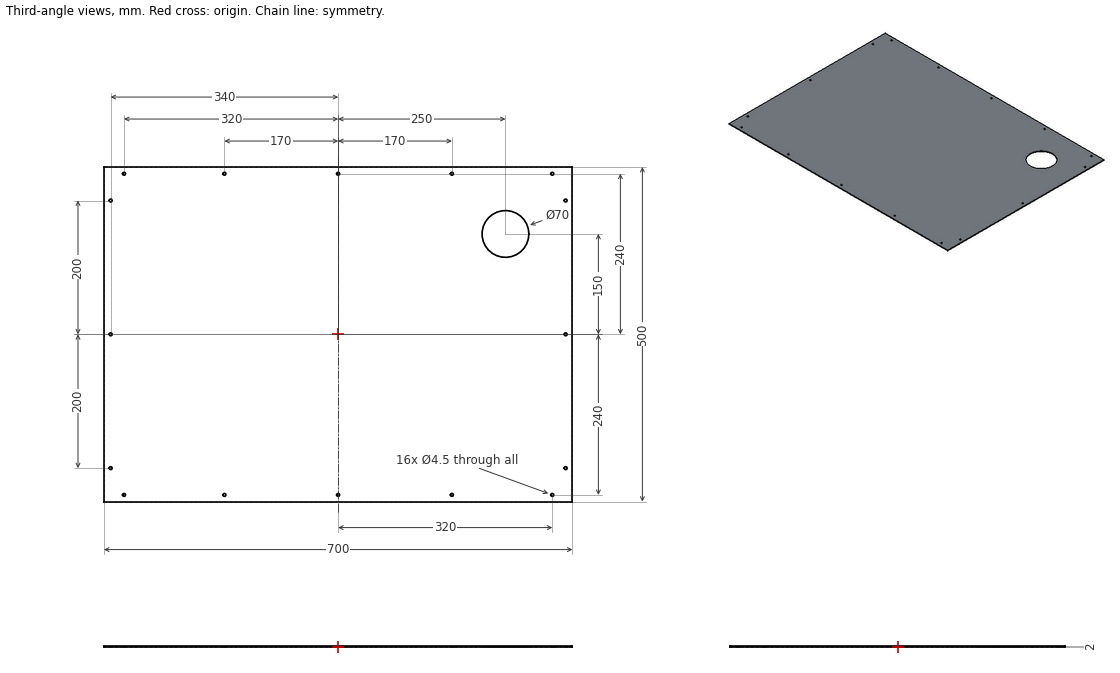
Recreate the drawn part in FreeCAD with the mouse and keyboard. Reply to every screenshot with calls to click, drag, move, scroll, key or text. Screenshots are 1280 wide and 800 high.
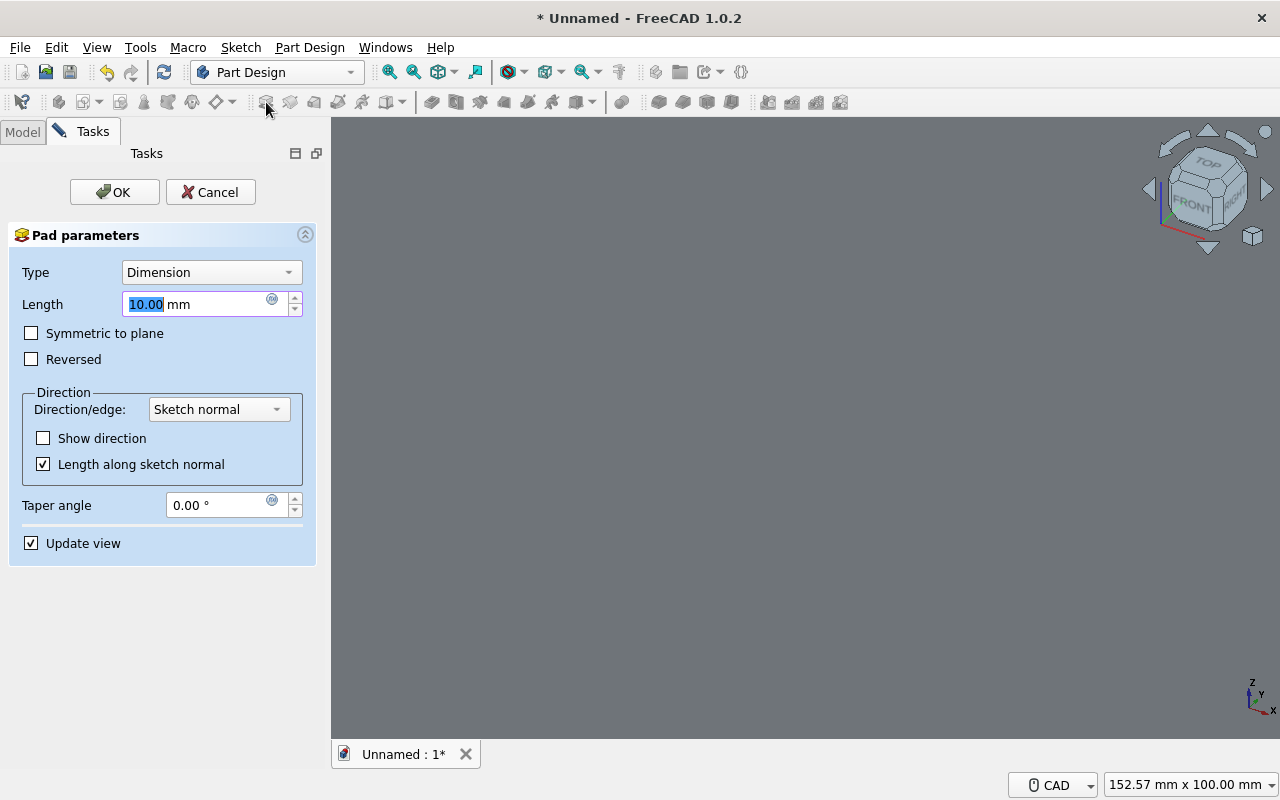
text(2)
key(Tab)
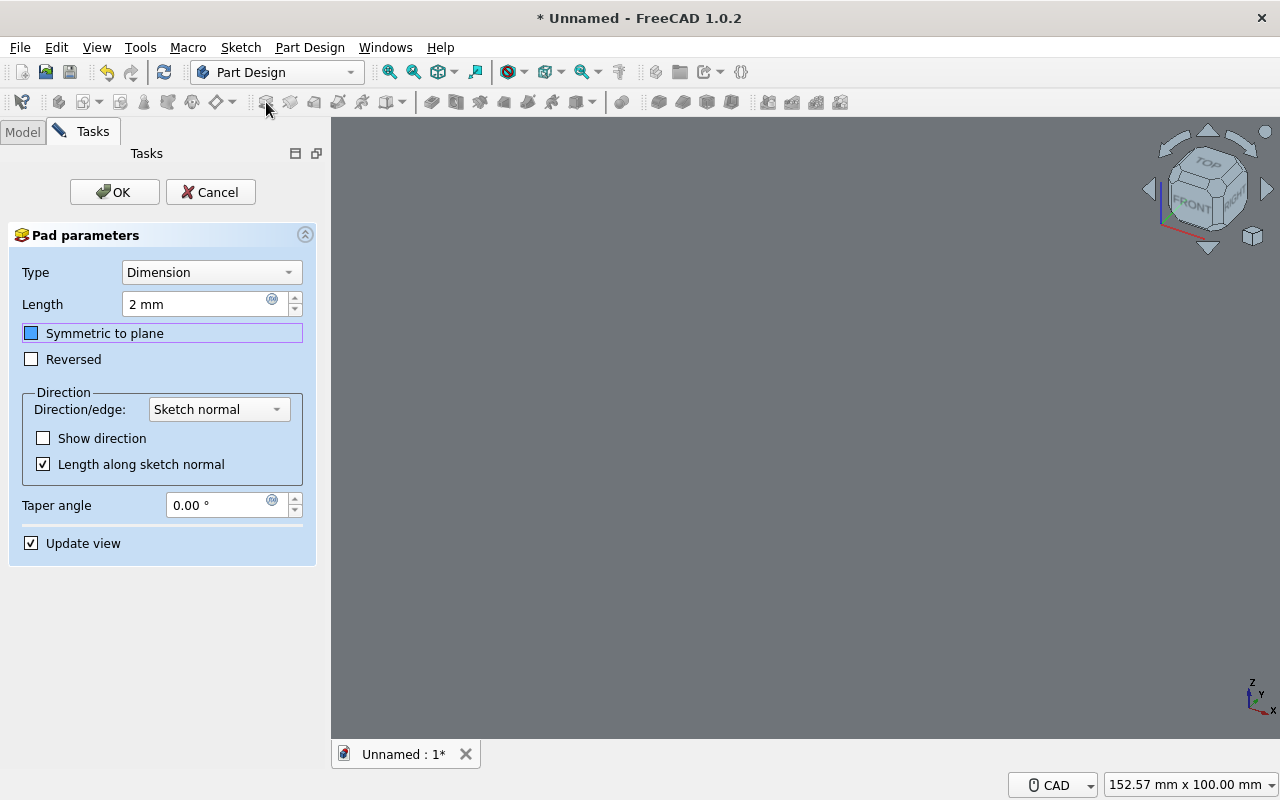
click(115, 192)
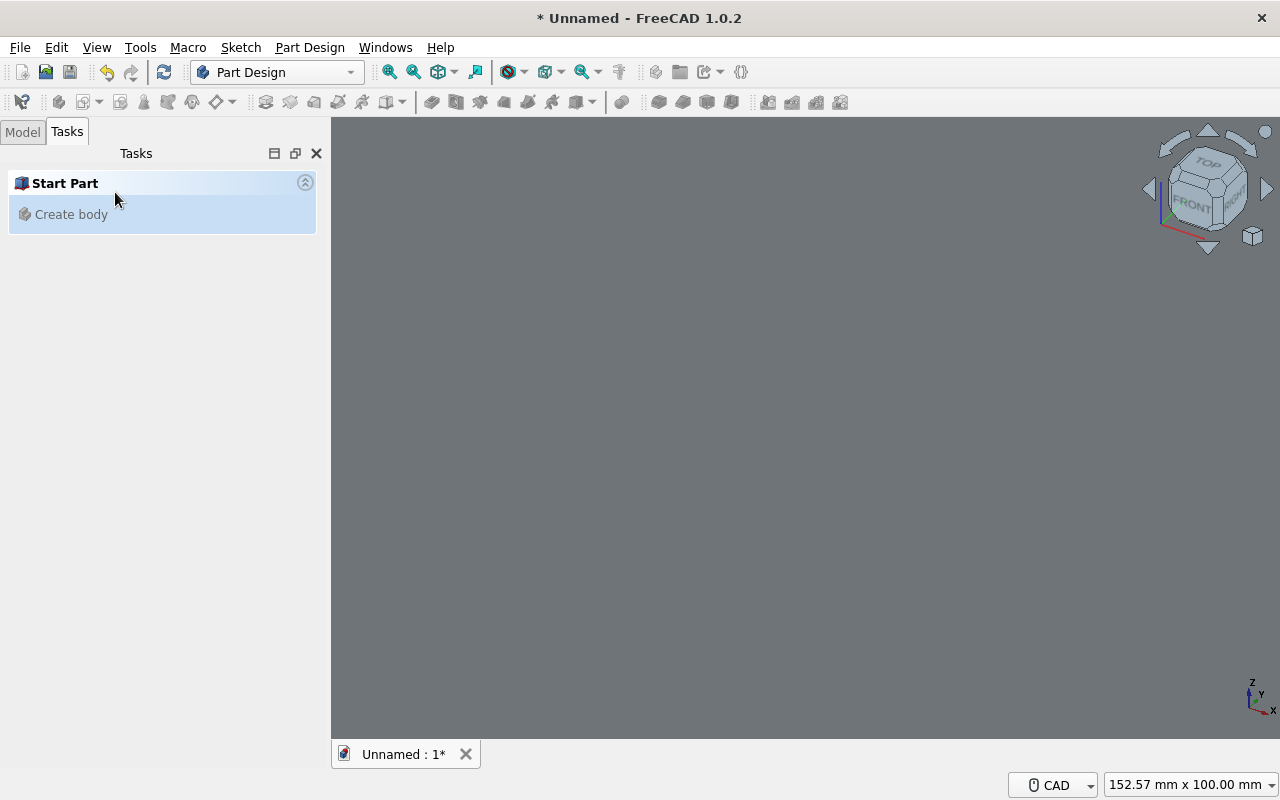
key(v)
key(f)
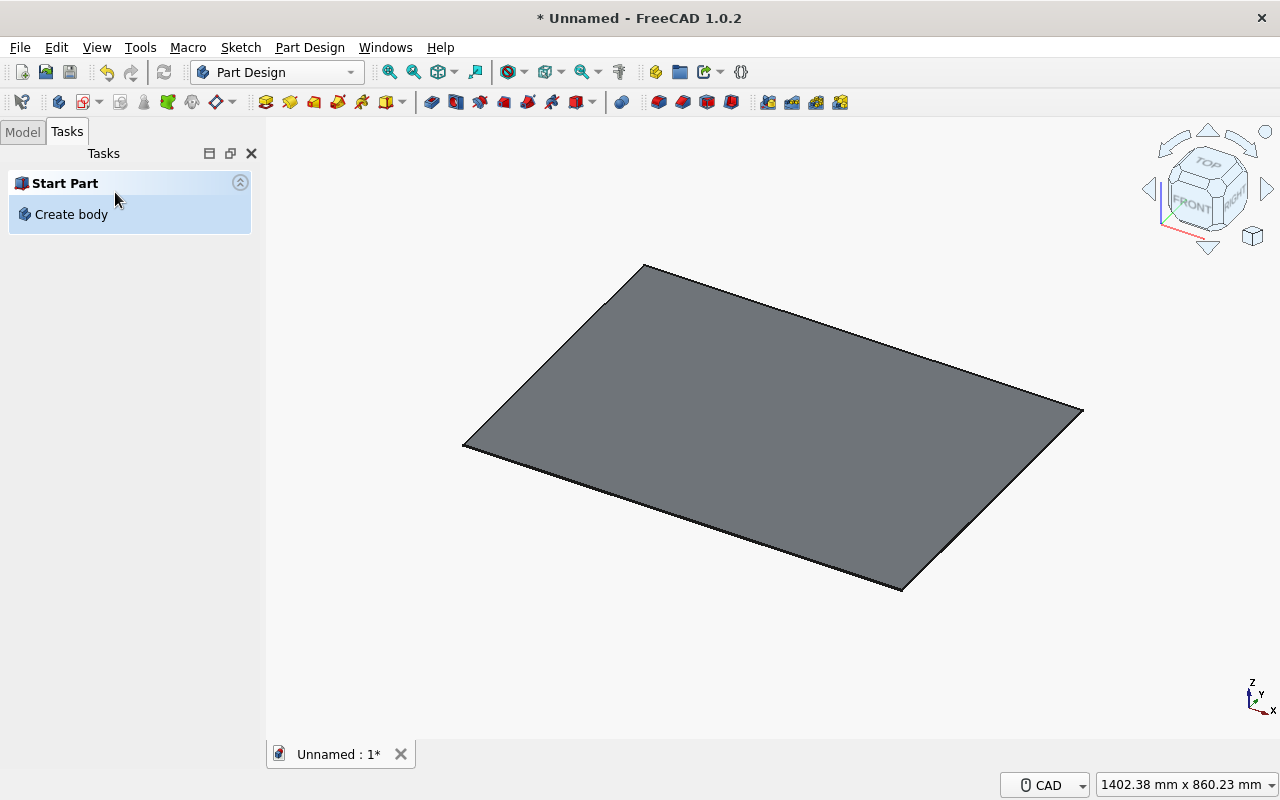
click(836, 447)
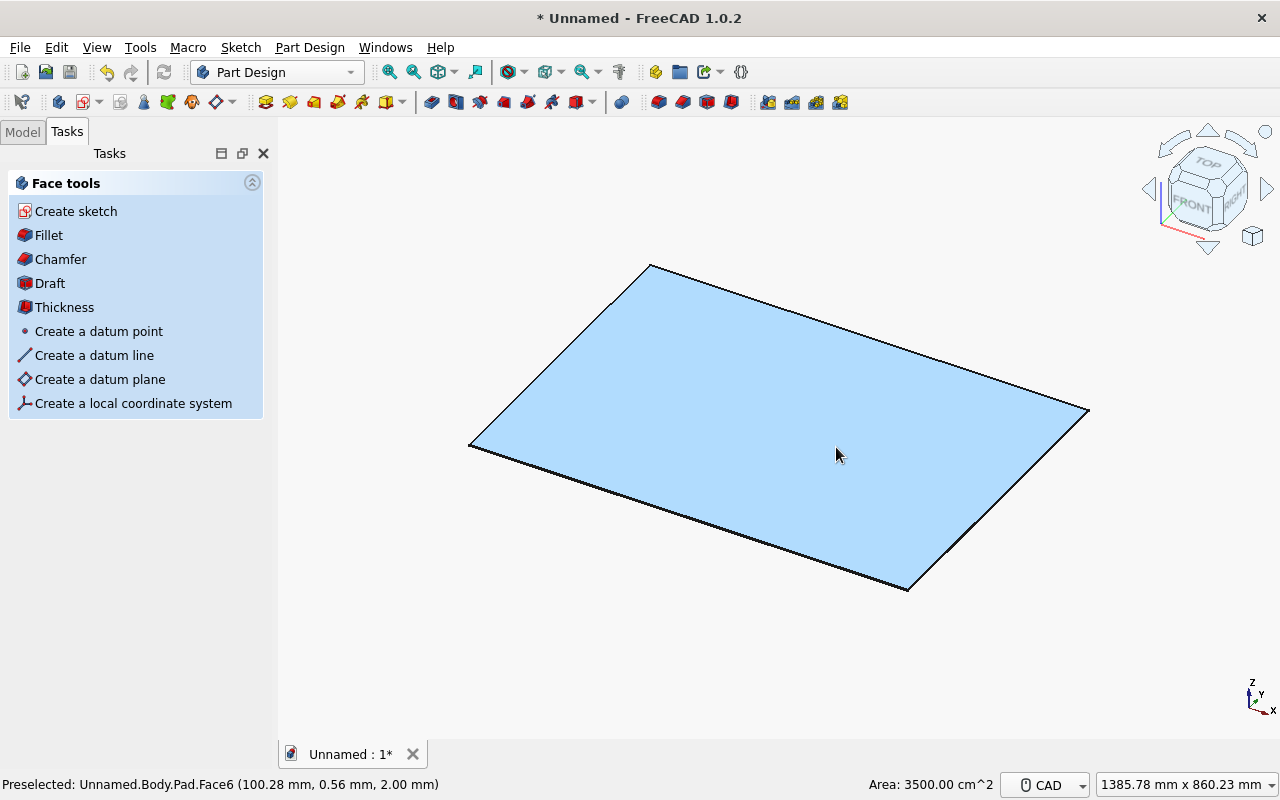
click(84, 102)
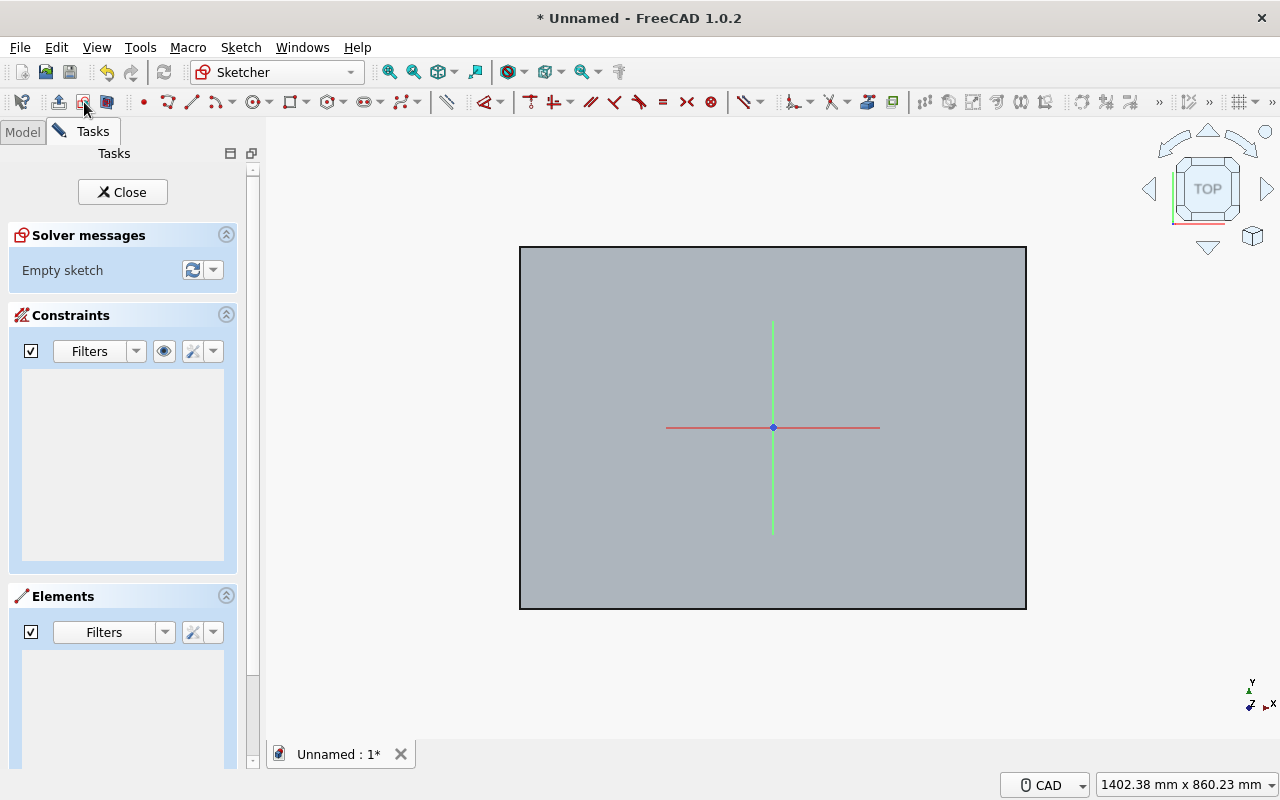
key(g)
key(c)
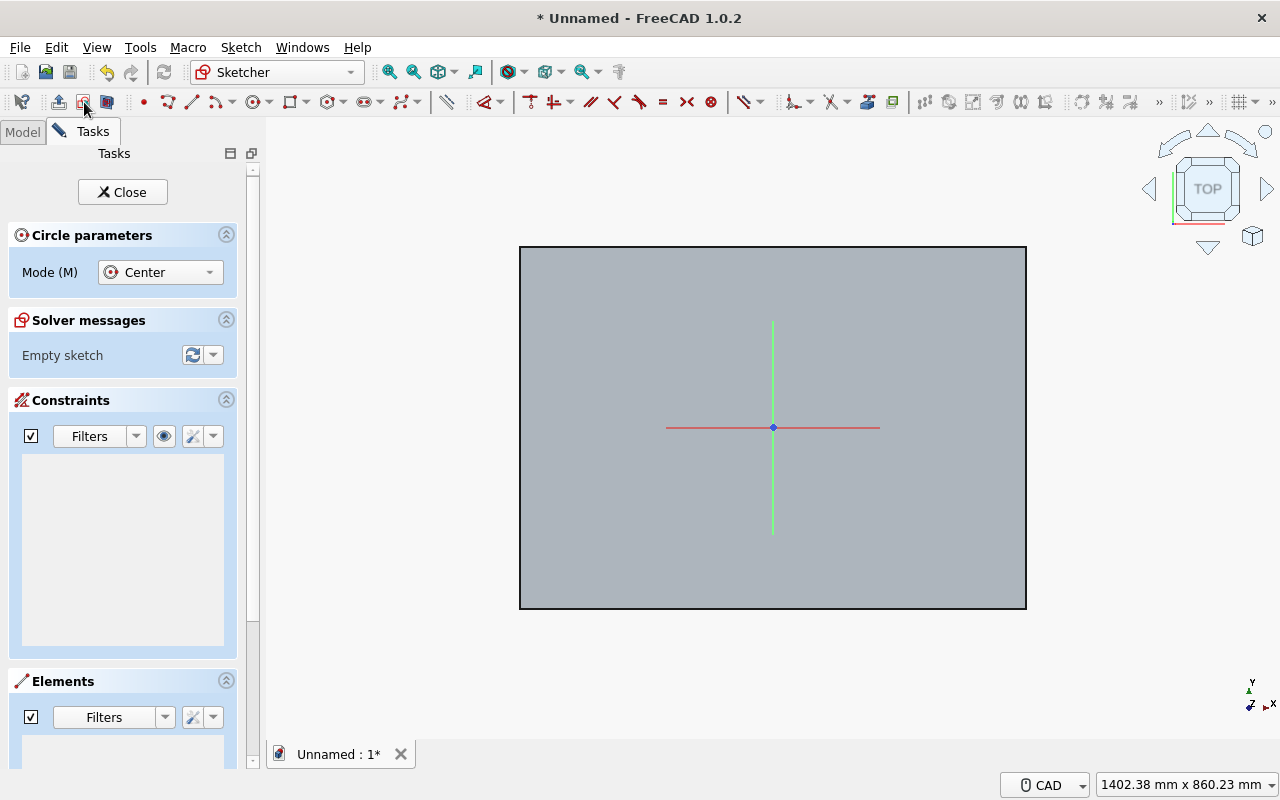
scroll(1004, 602, up, 14)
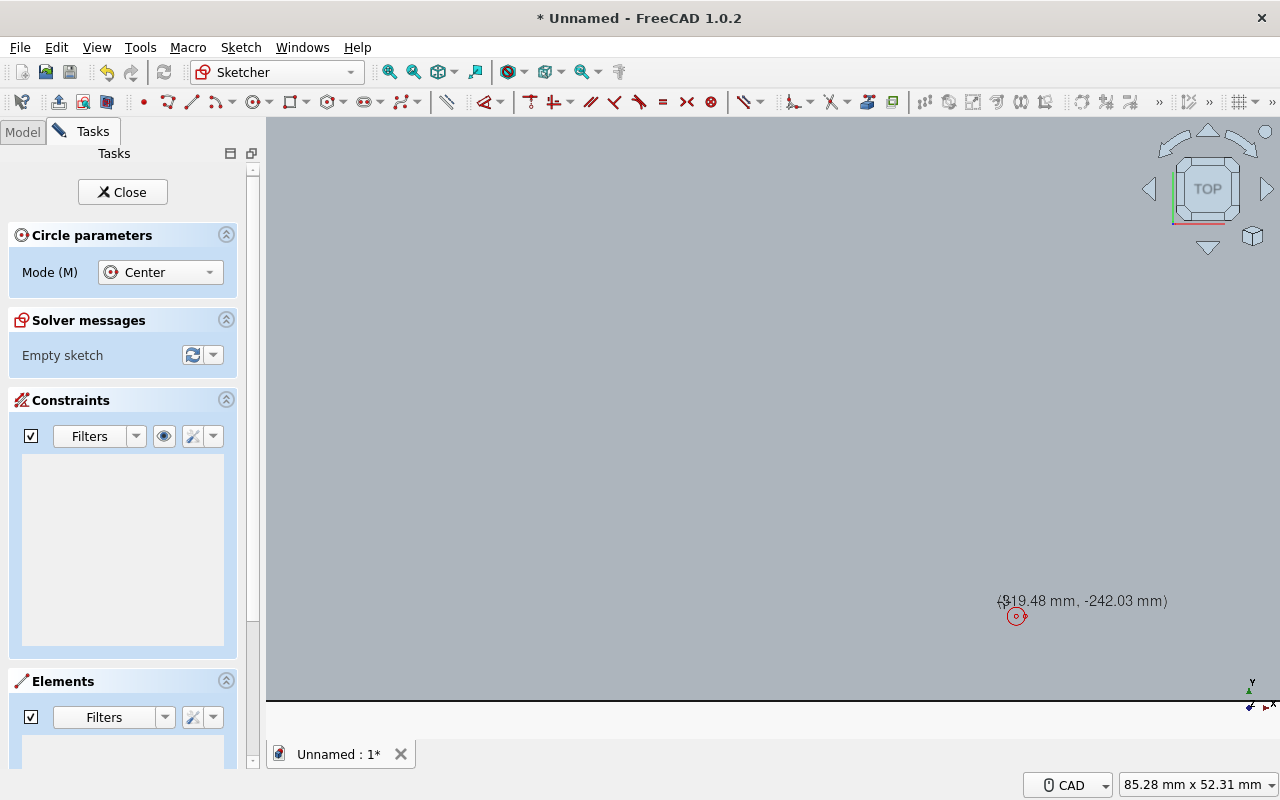
scroll(986, 645, down, 13)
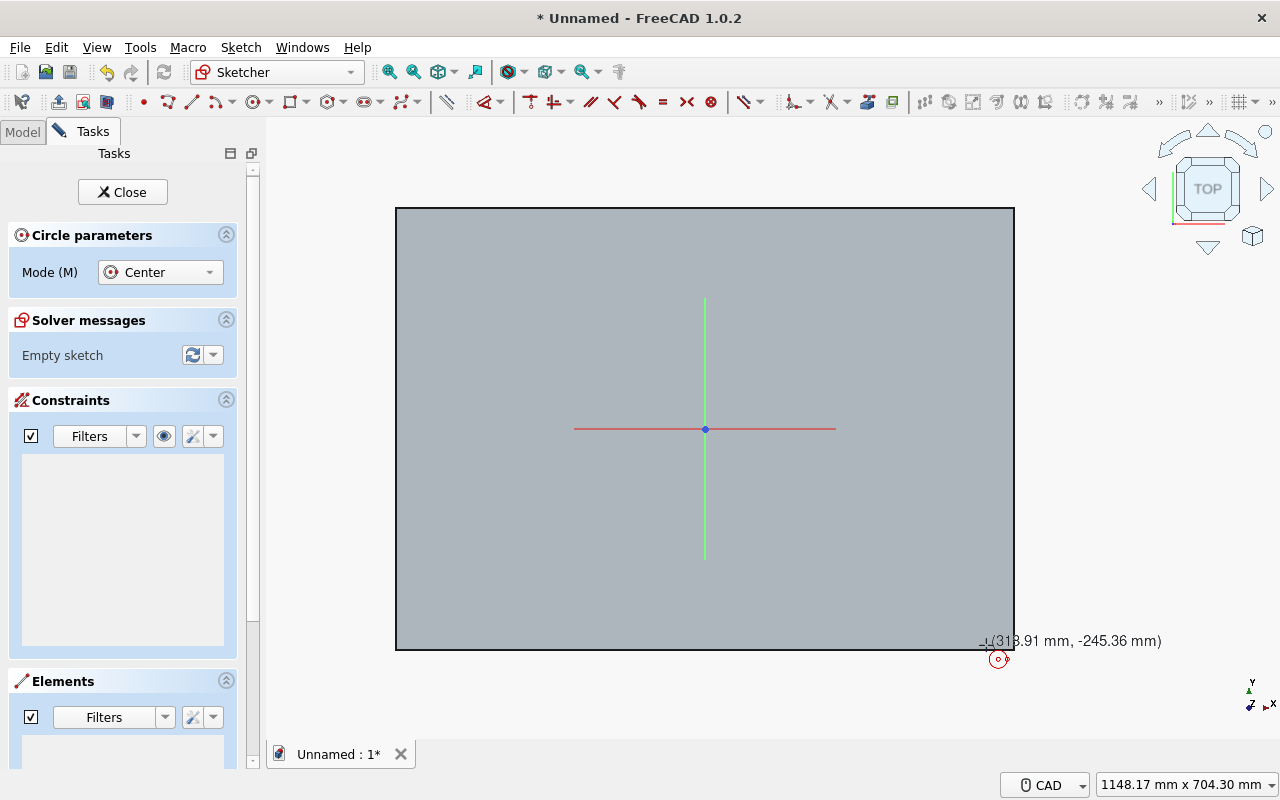
click(988, 641)
move(989, 640)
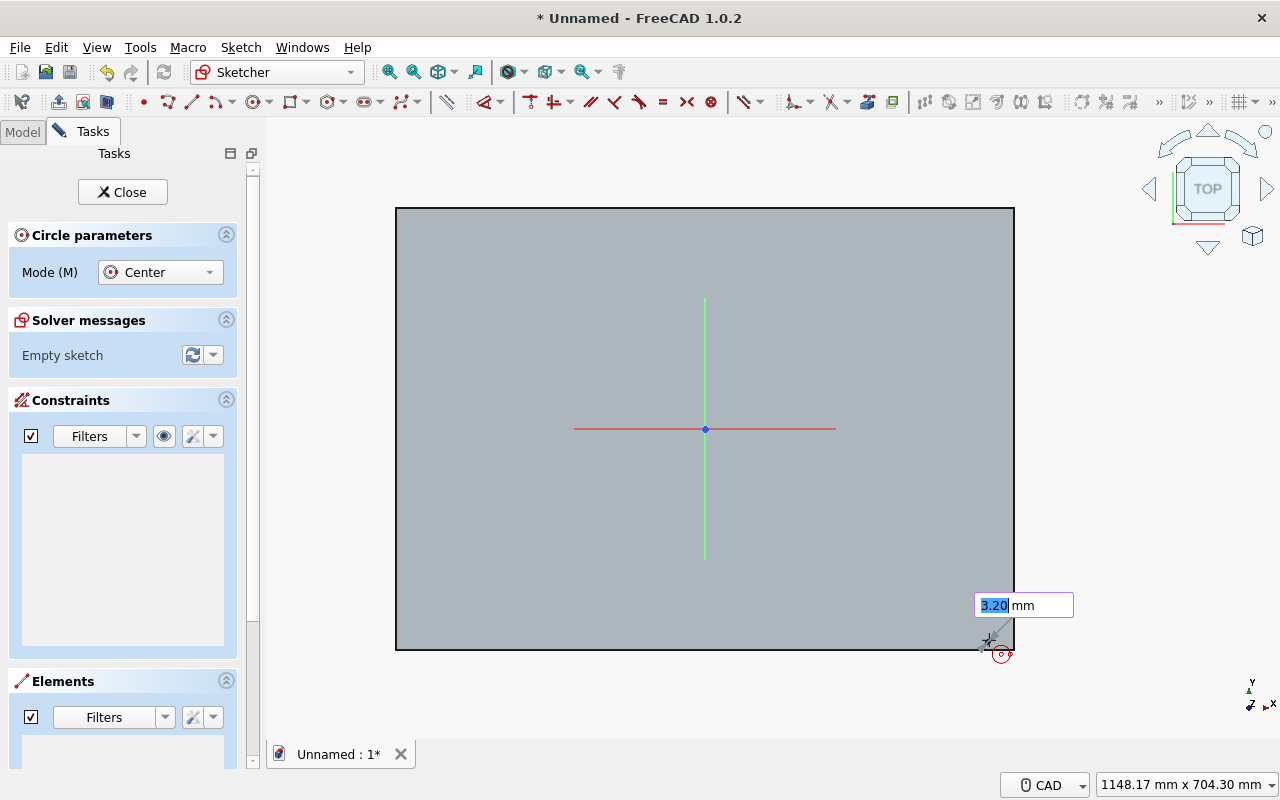
text(4.5)
key(Return)